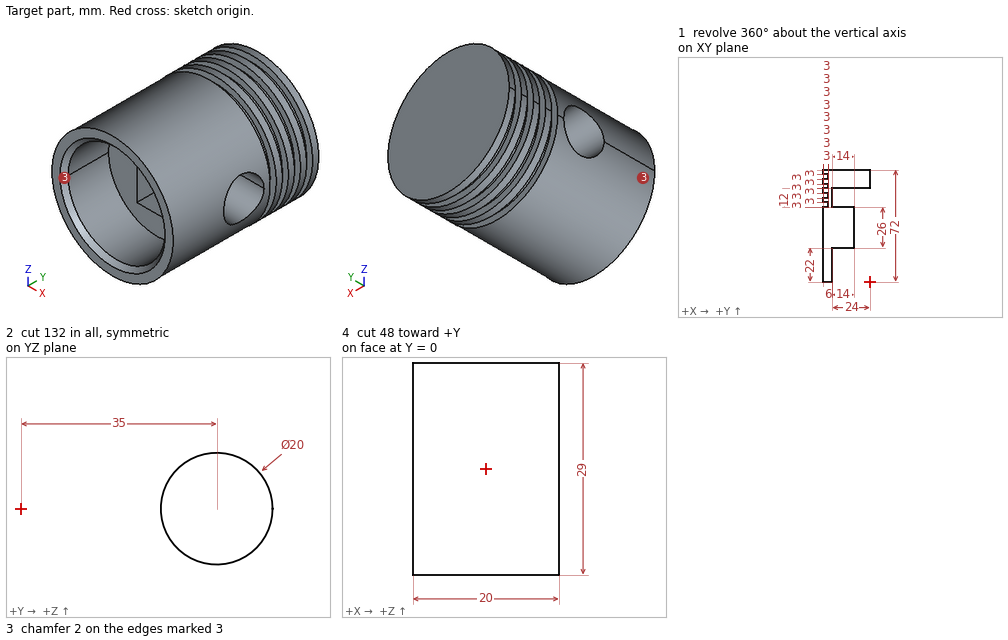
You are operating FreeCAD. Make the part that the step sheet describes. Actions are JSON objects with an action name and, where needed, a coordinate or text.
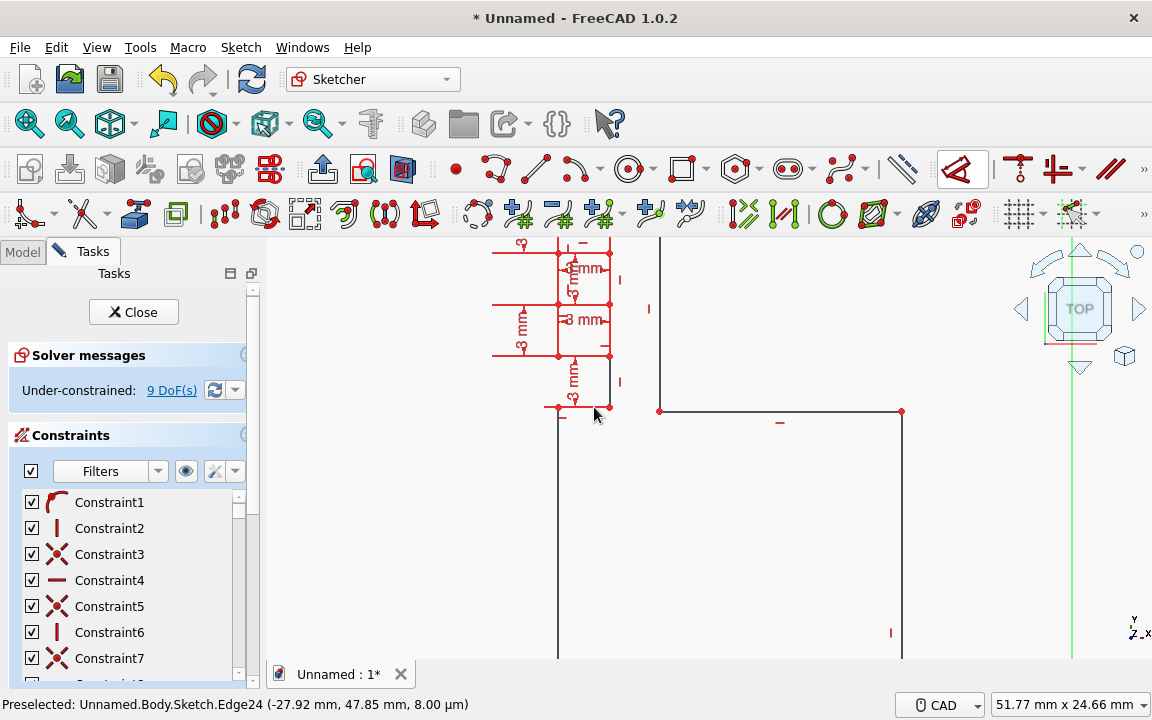
{"action": "key", "text": "l"}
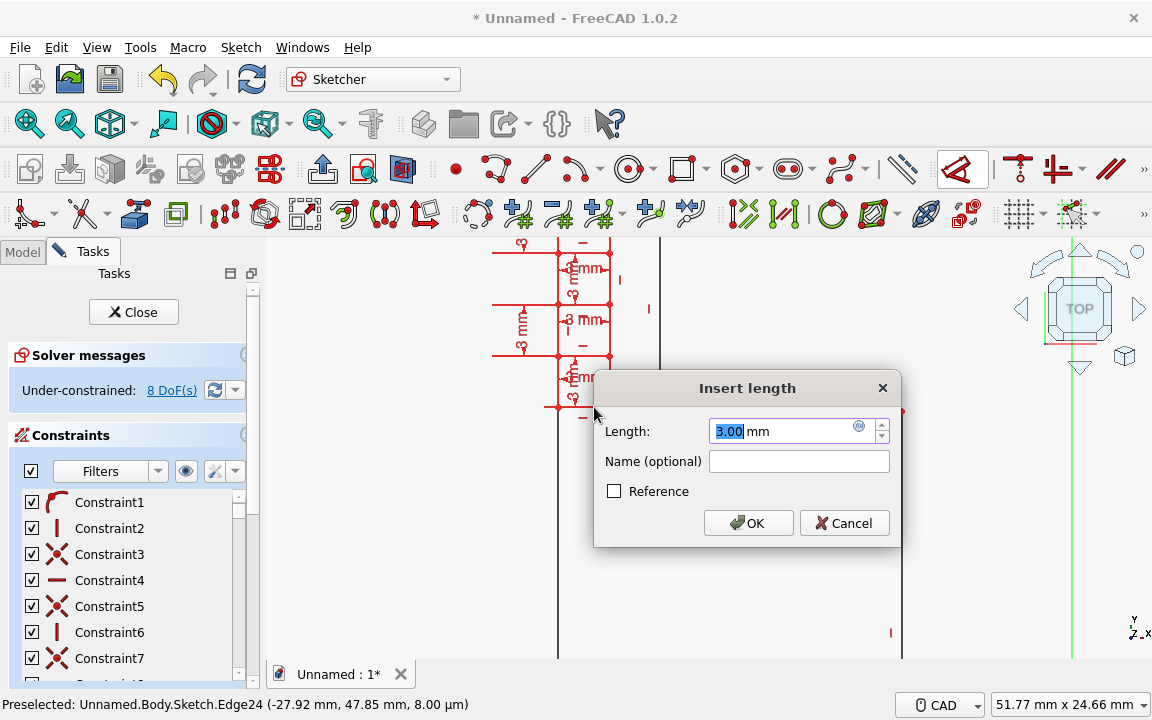
{"action": "type", "text": "3"}
{"action": "key", "text": "Return"}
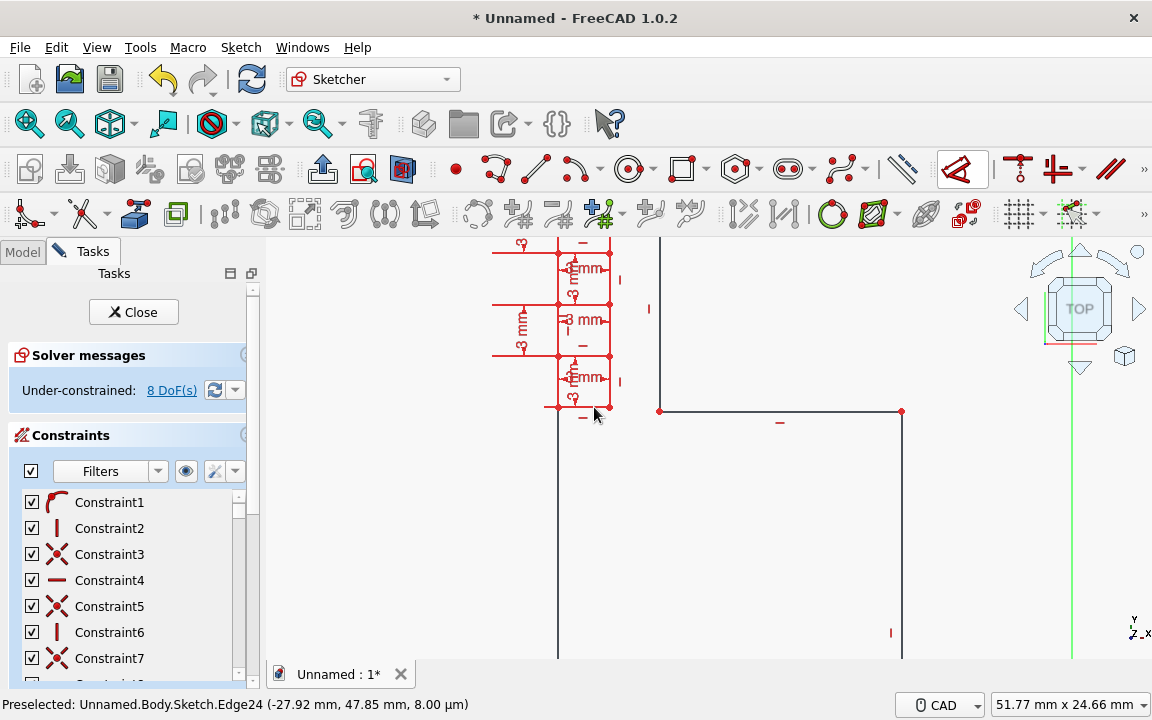
{"action": "scroll", "coordinate": [596, 407], "scroll_direction": "down", "scroll_amount": 8}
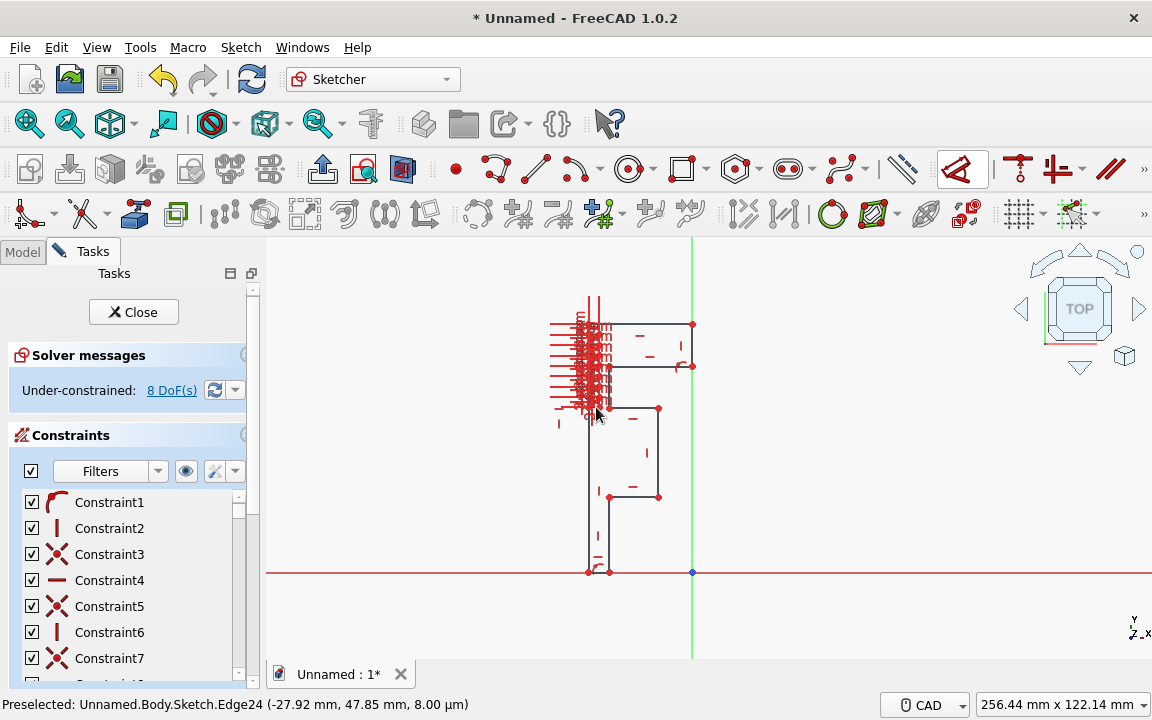
{"action": "scroll", "coordinate": [595, 573], "scroll_direction": "up", "scroll_amount": 5}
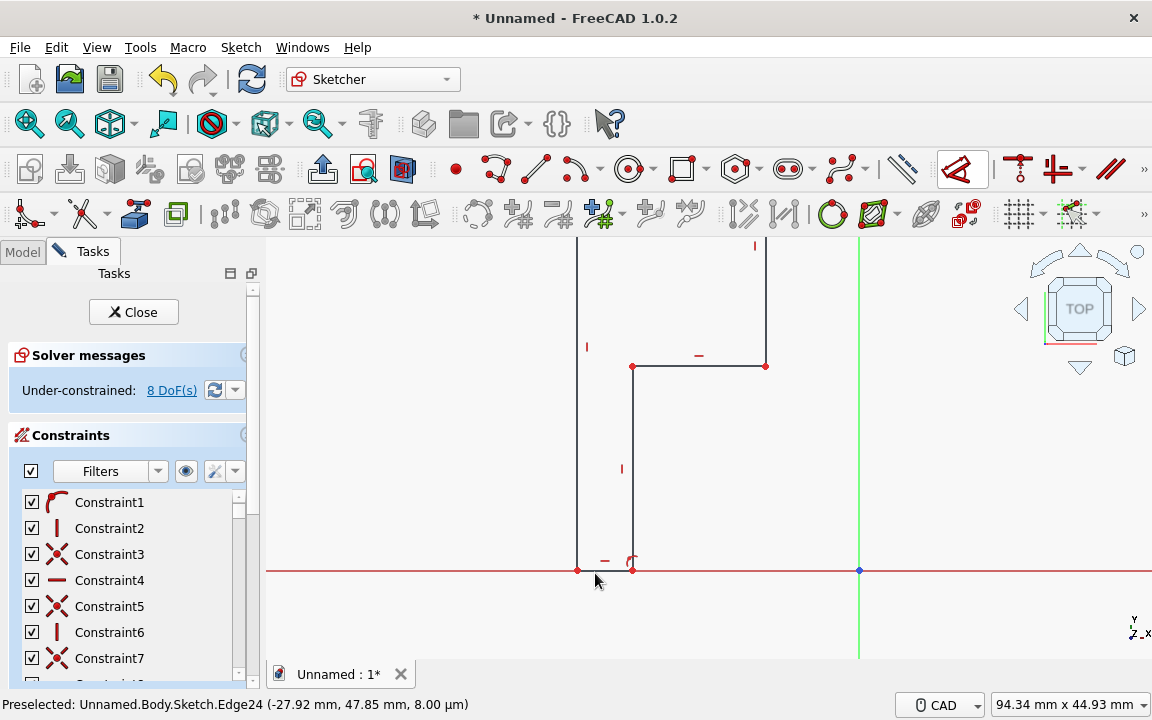
{"action": "left_click", "coordinate": [594, 571]}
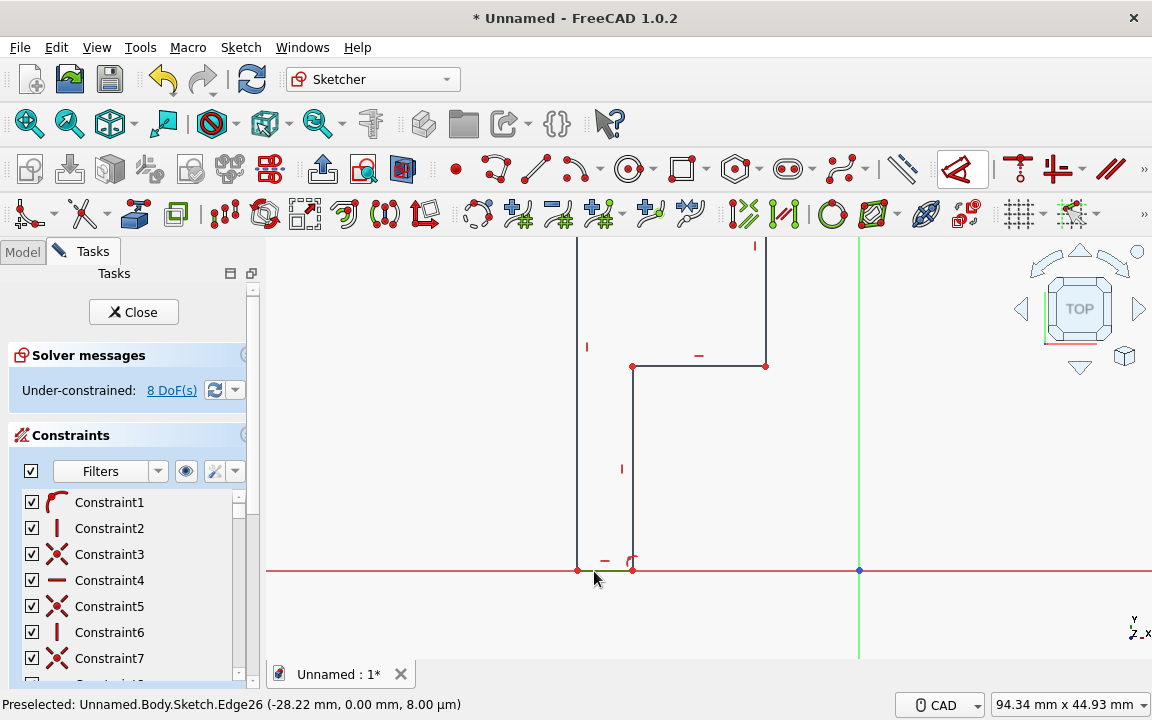
{"action": "key", "text": "l"}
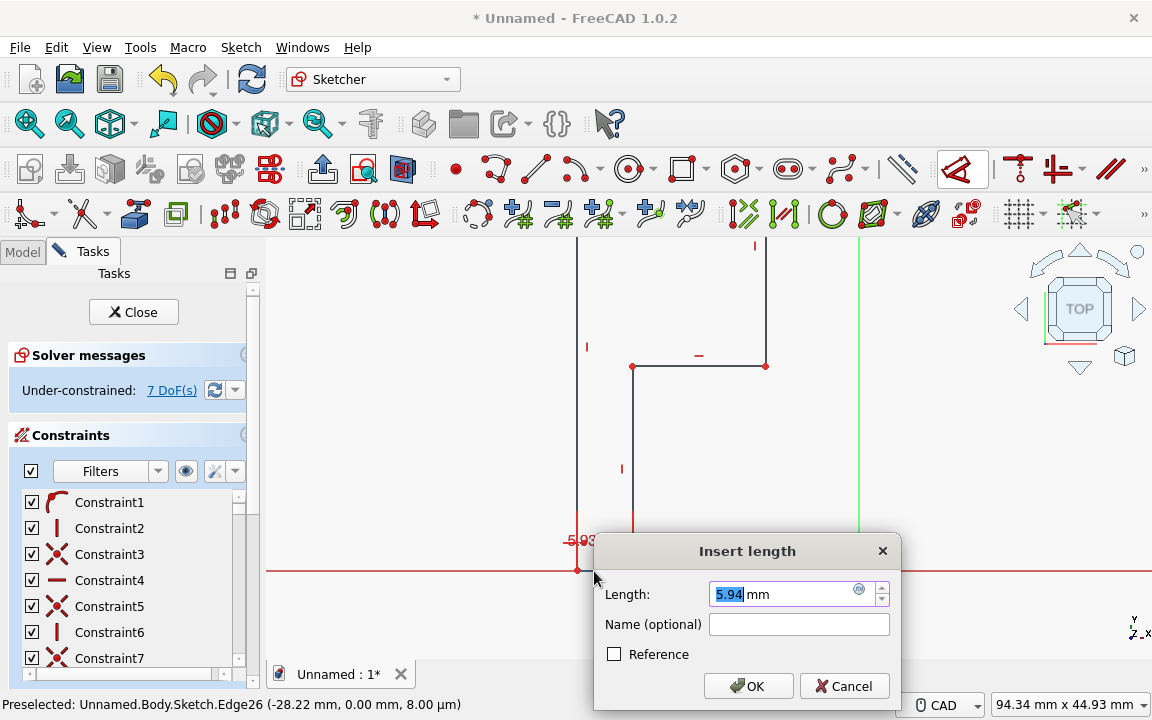
{"action": "type", "text": "6"}
{"action": "key", "text": "Return"}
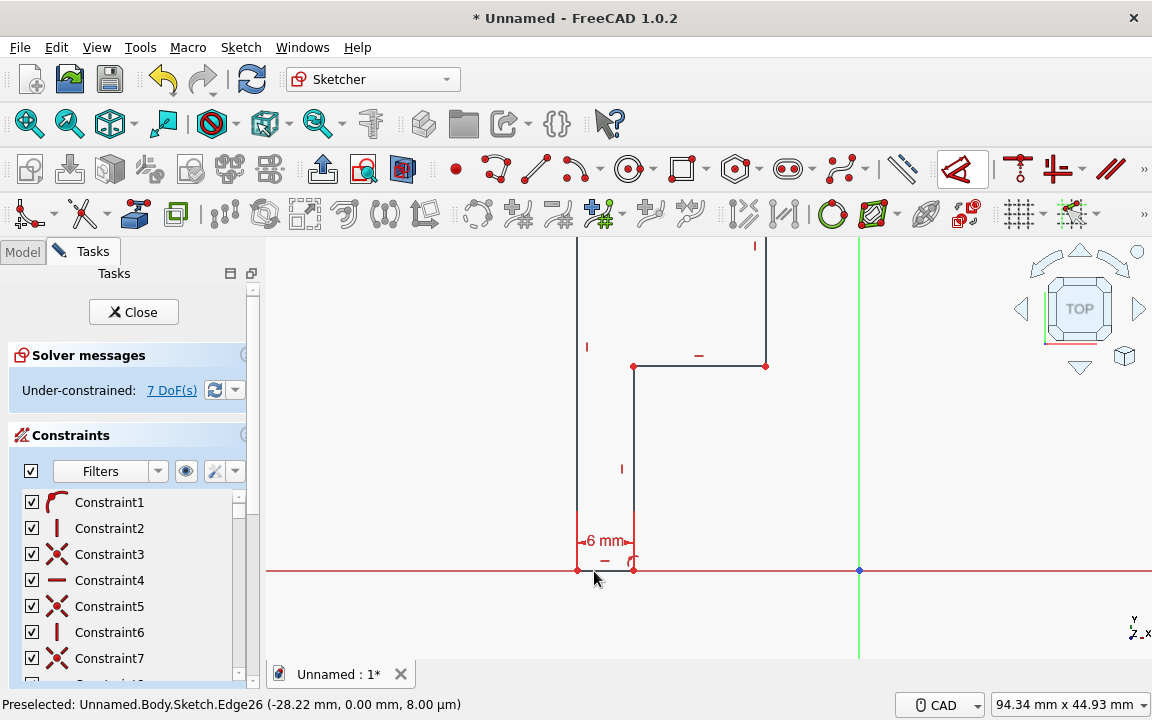
{"action": "left_click", "coordinate": [634, 509]}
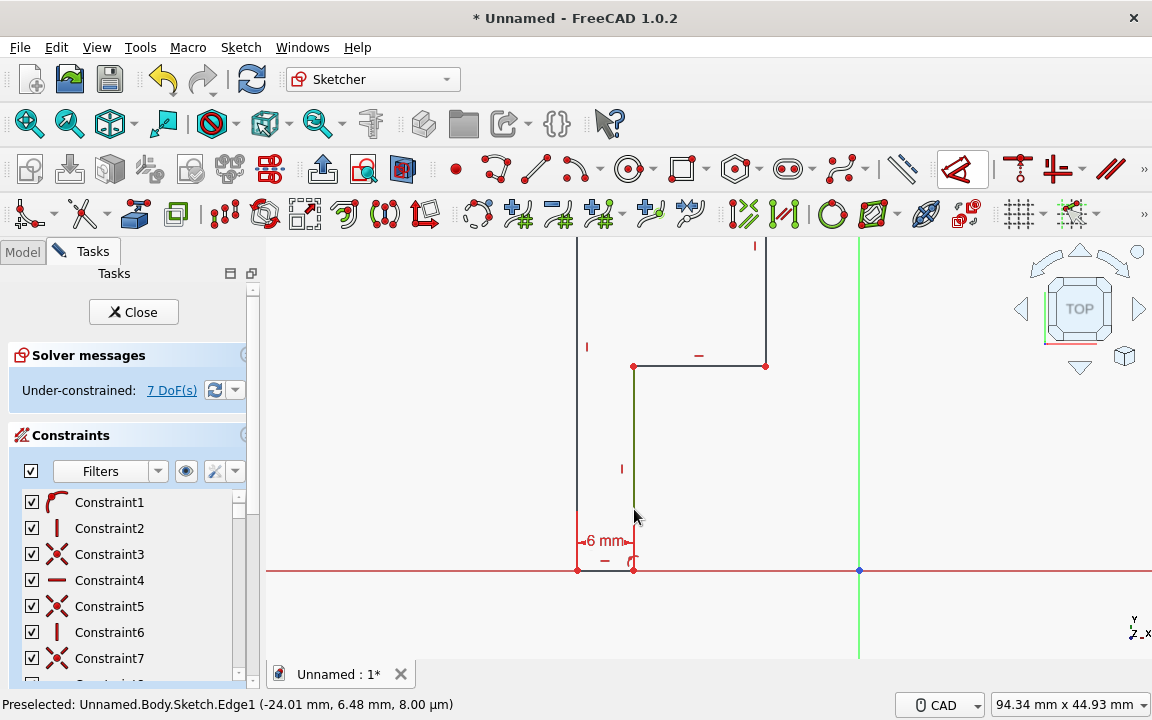
{"action": "key", "text": "i"}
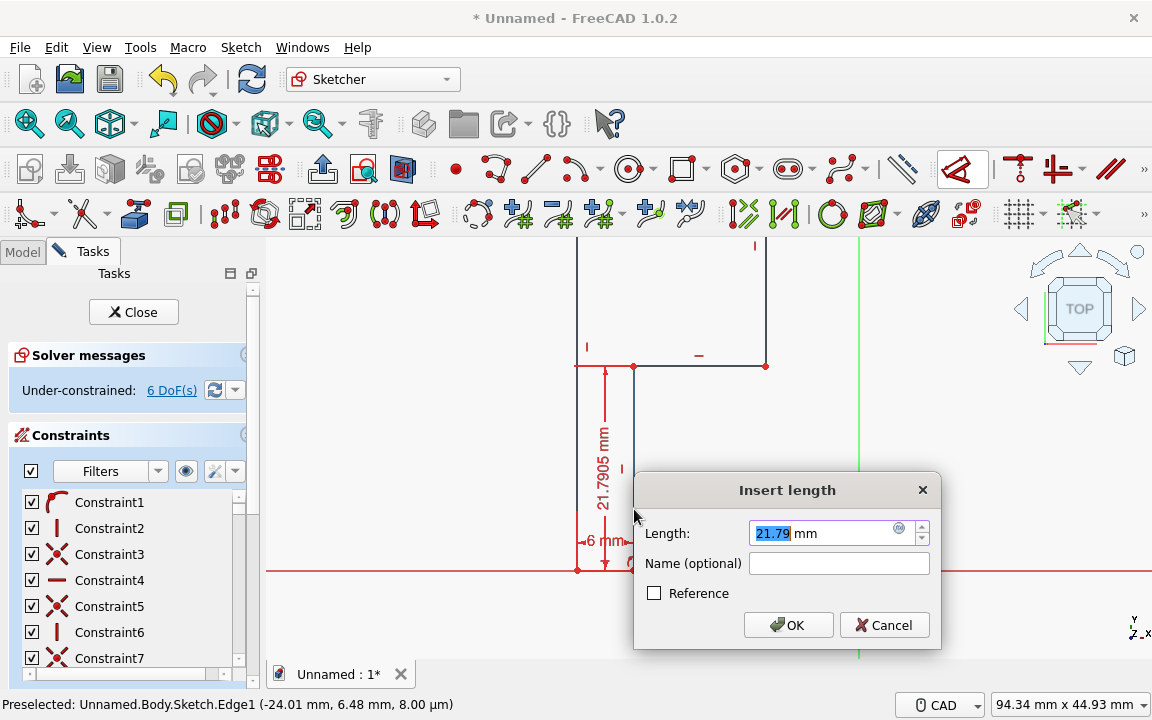
{"action": "type", "text": "22"}
{"action": "key", "text": "Return"}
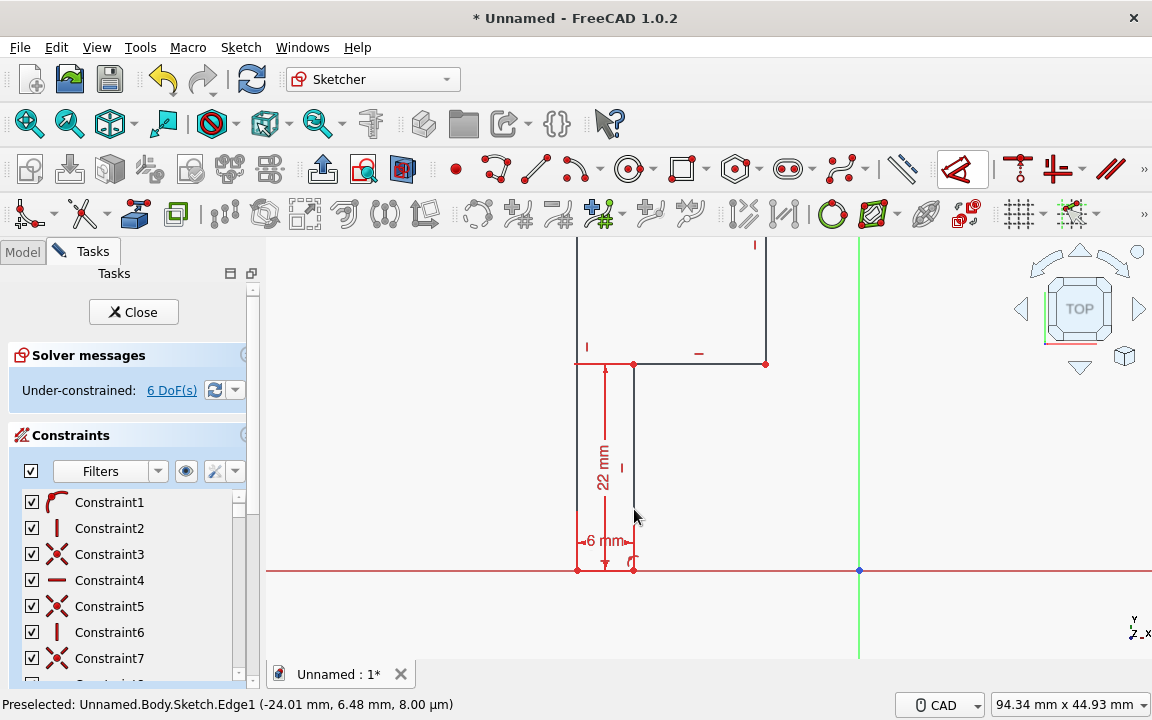
{"action": "left_click", "coordinate": [673, 364]}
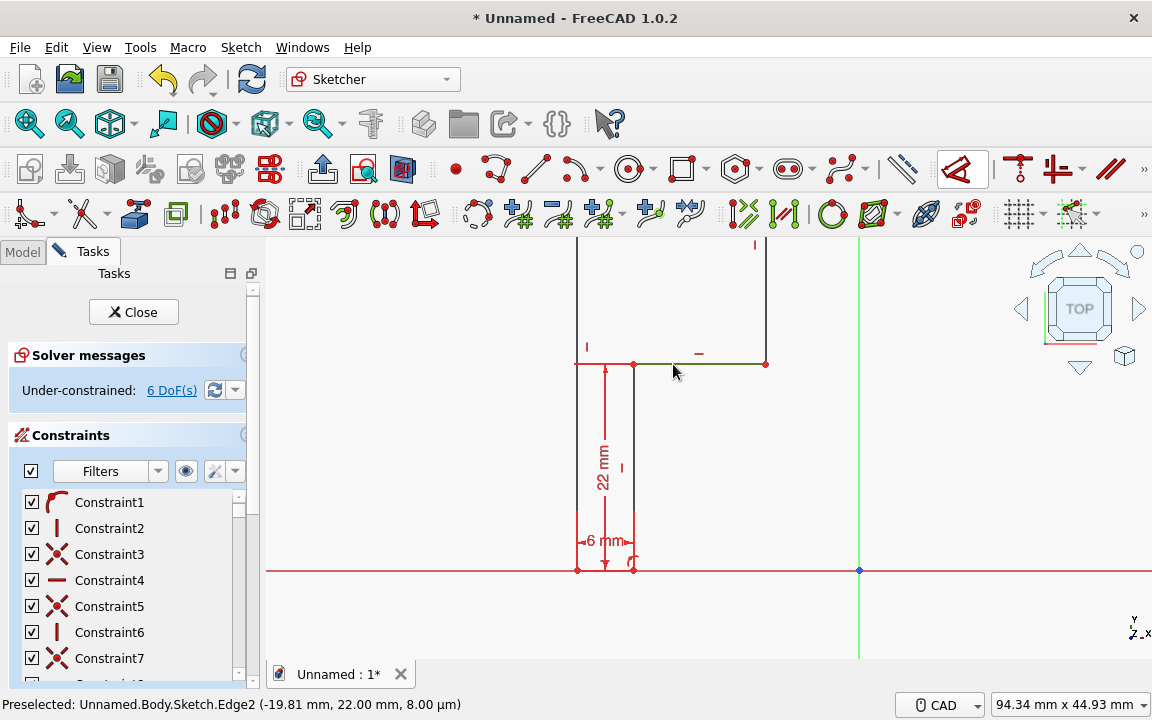
{"action": "key", "text": "l"}